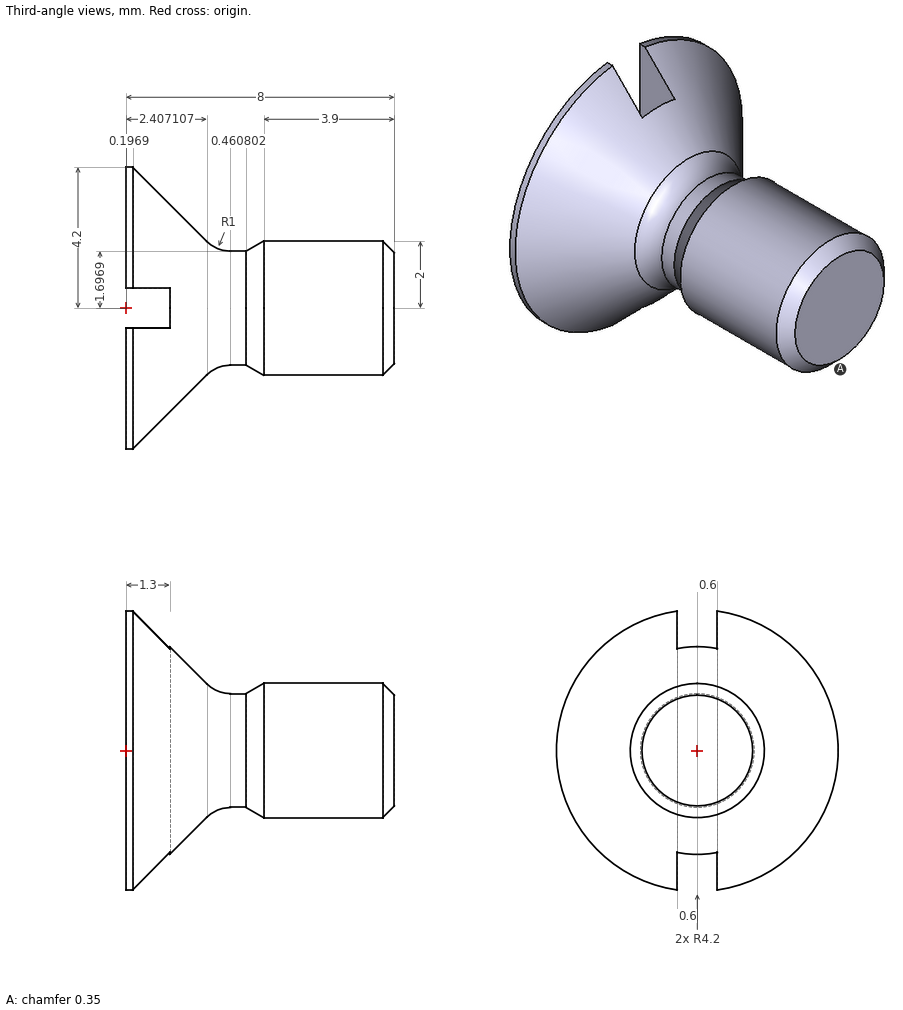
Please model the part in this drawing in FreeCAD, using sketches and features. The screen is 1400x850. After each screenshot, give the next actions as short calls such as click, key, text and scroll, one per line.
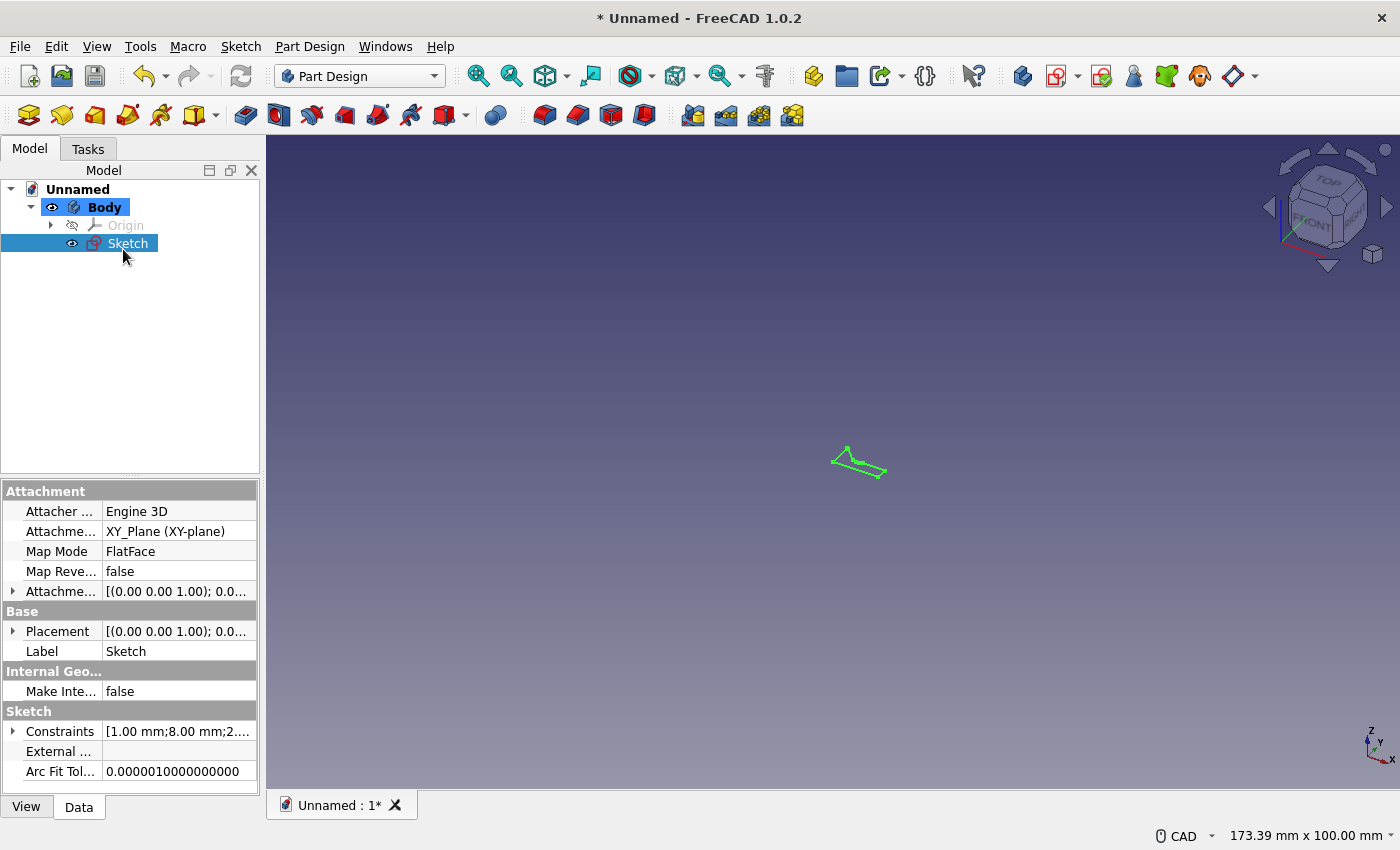
click(62, 116)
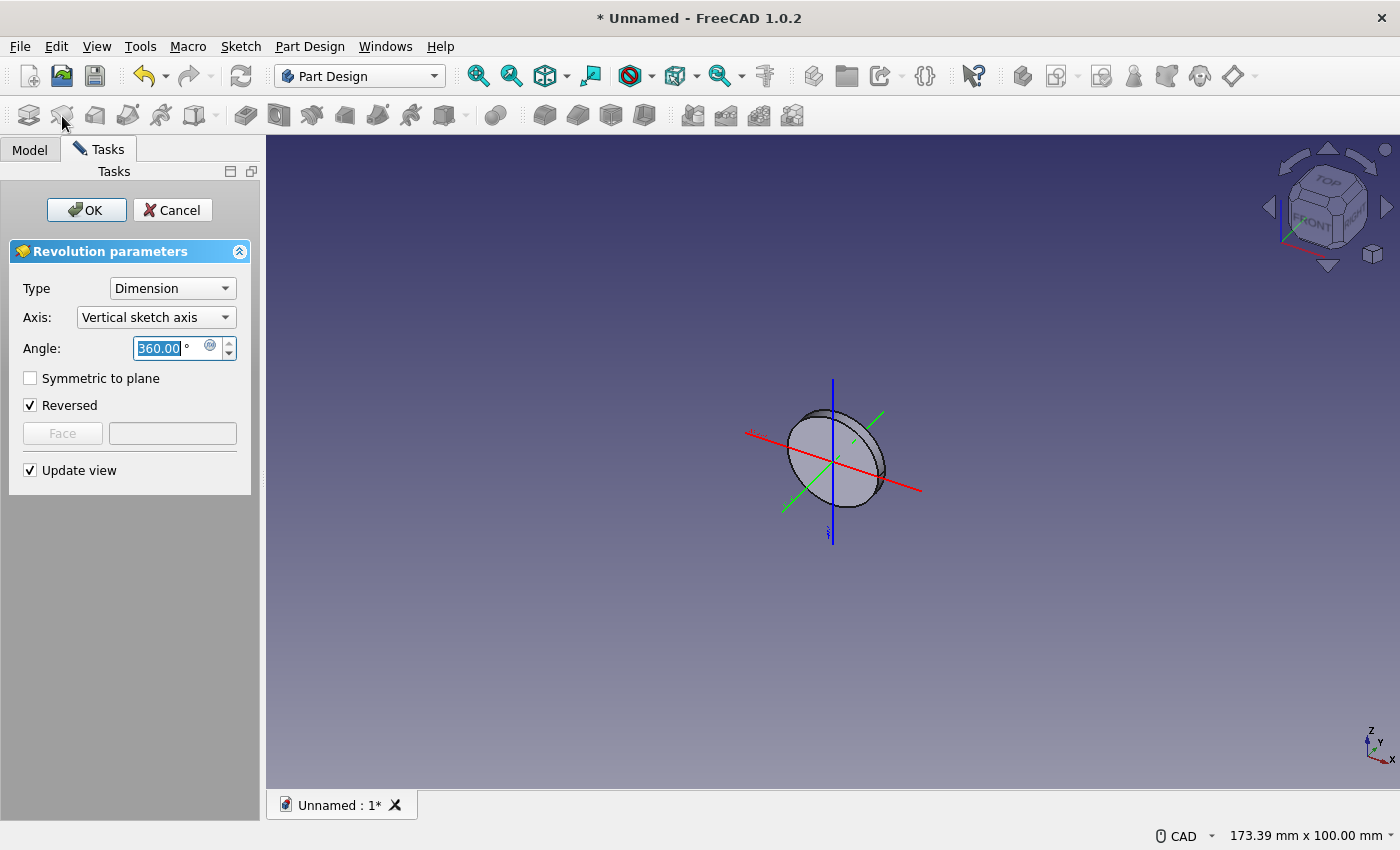
click(157, 318)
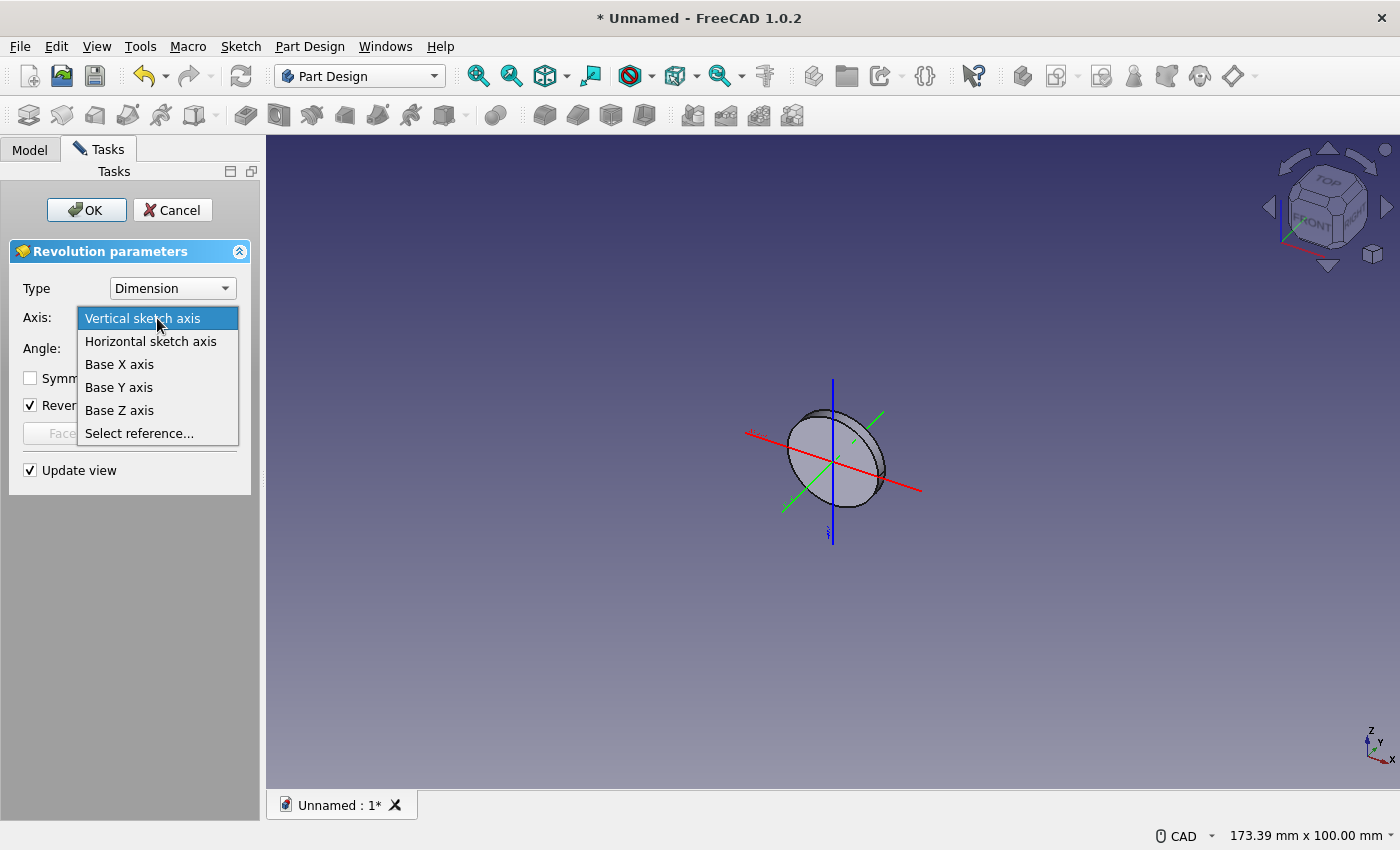
click(156, 342)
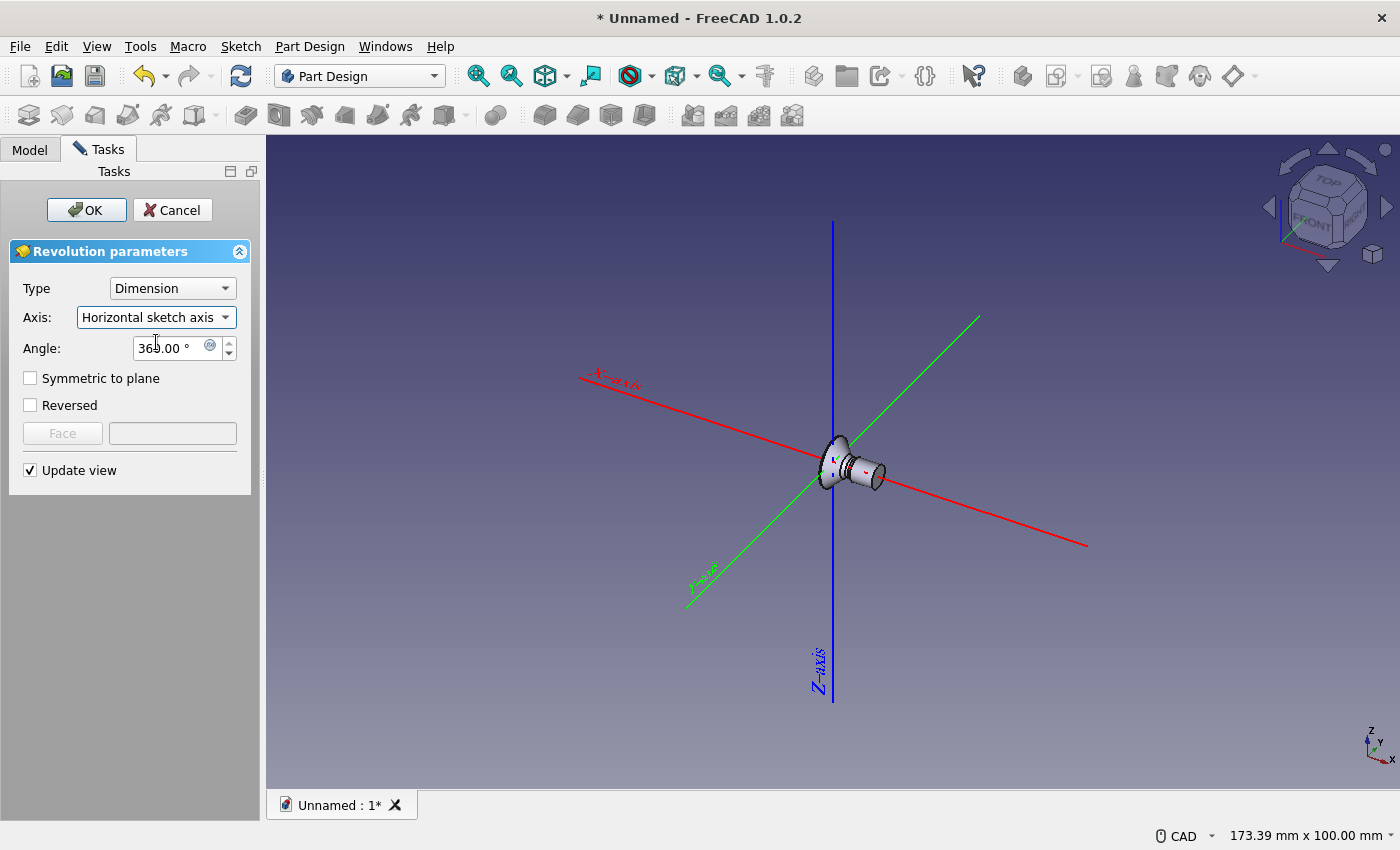
click(87, 210)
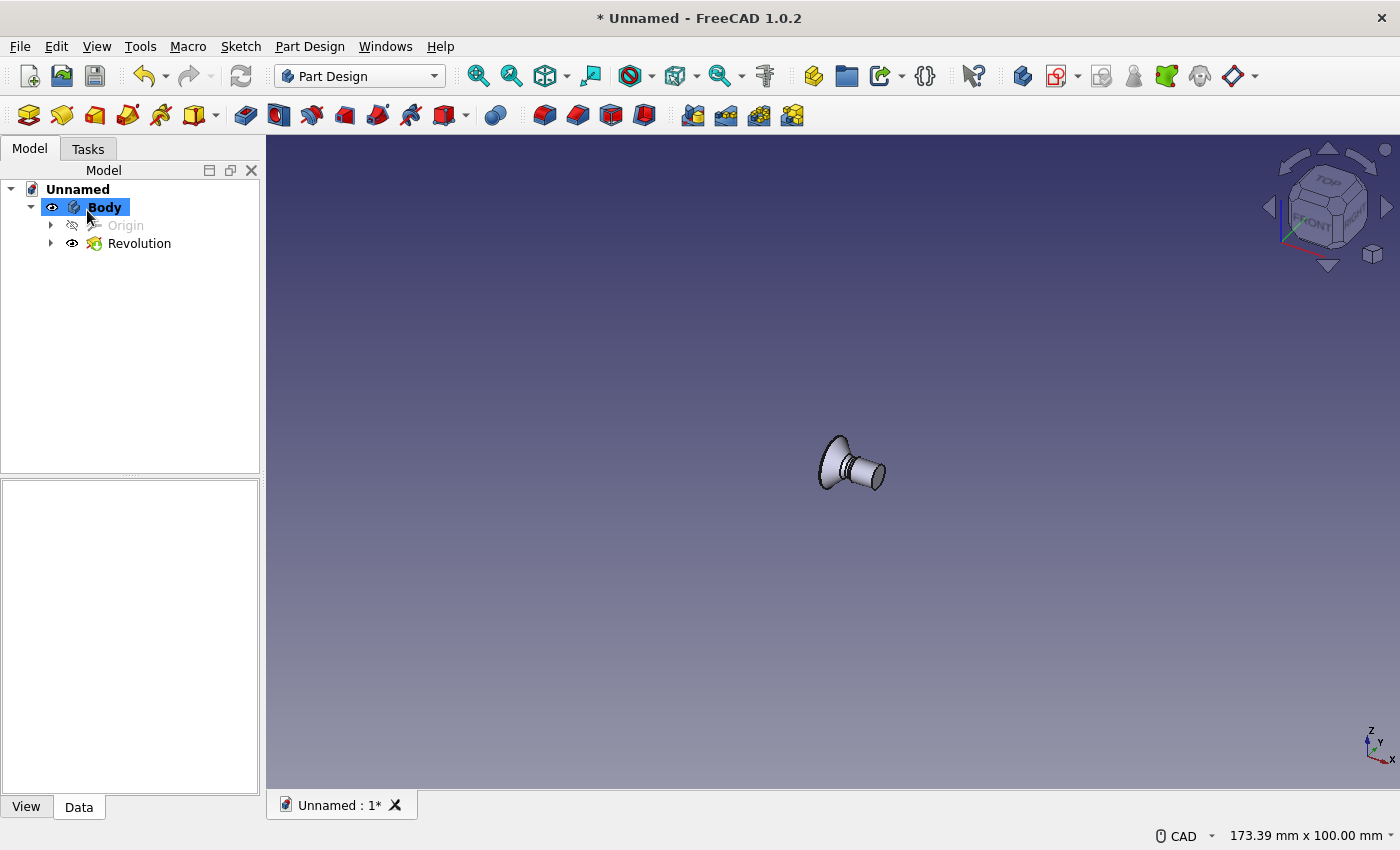
key(v)
key(f)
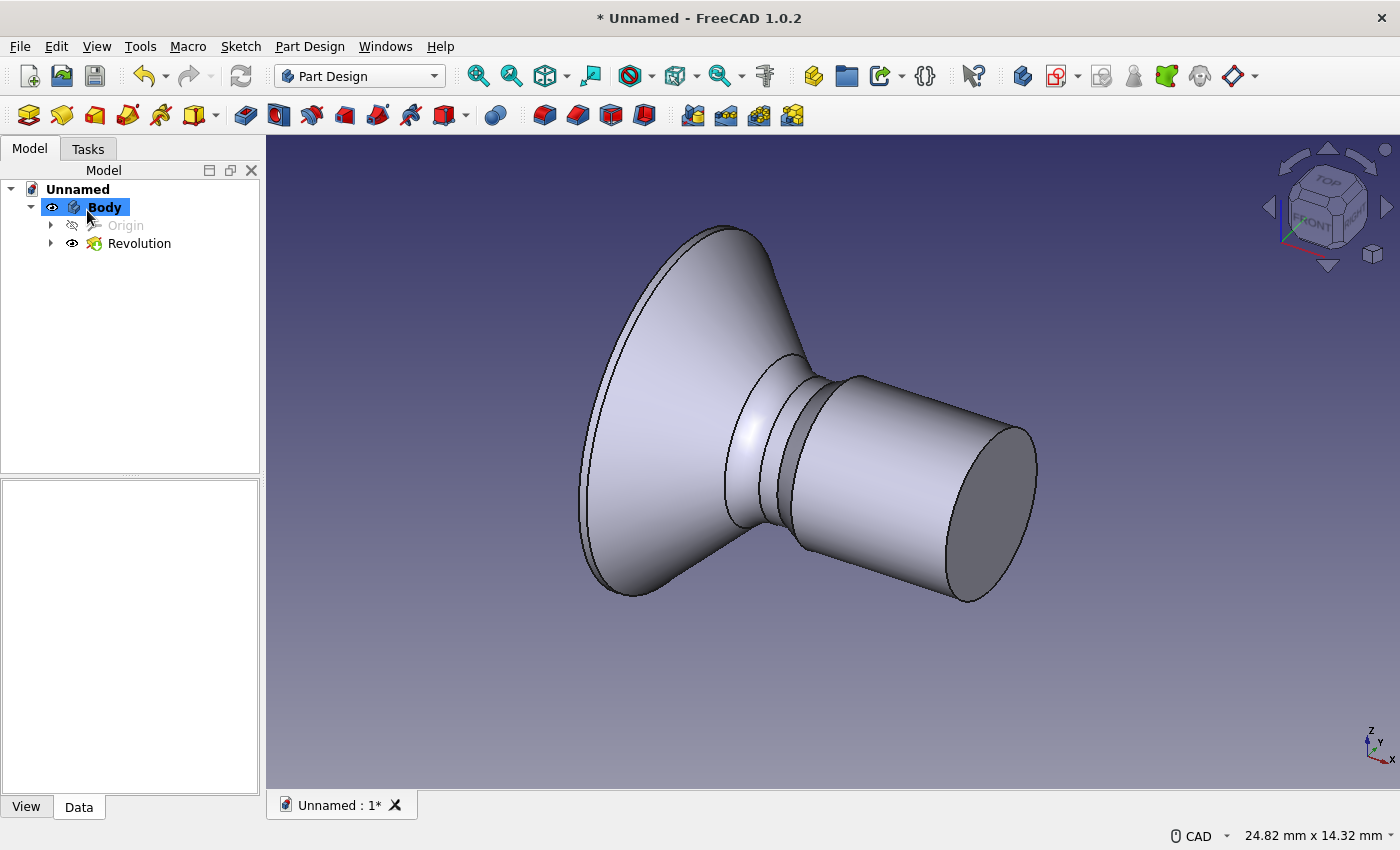
click(945, 559)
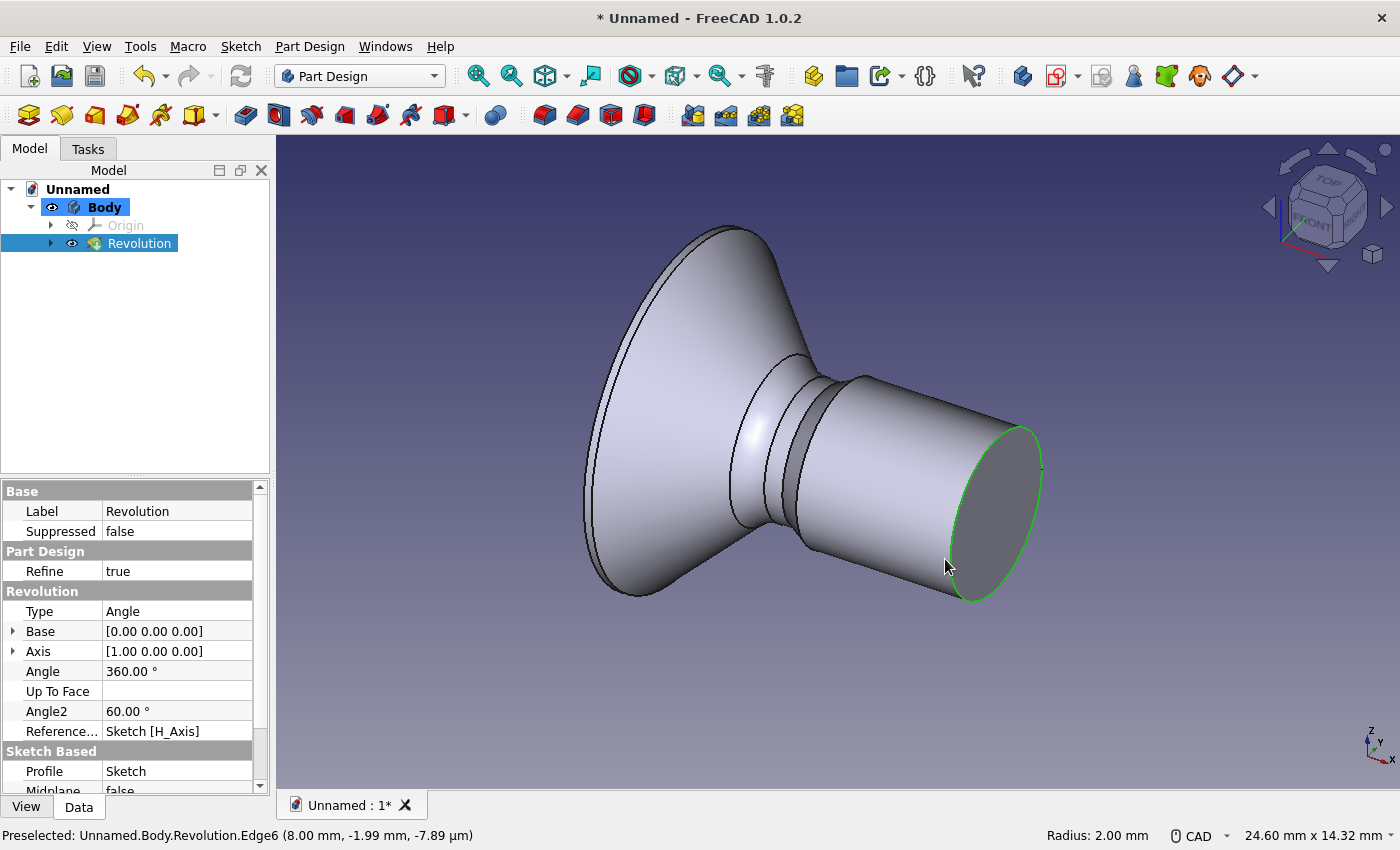
click(578, 116)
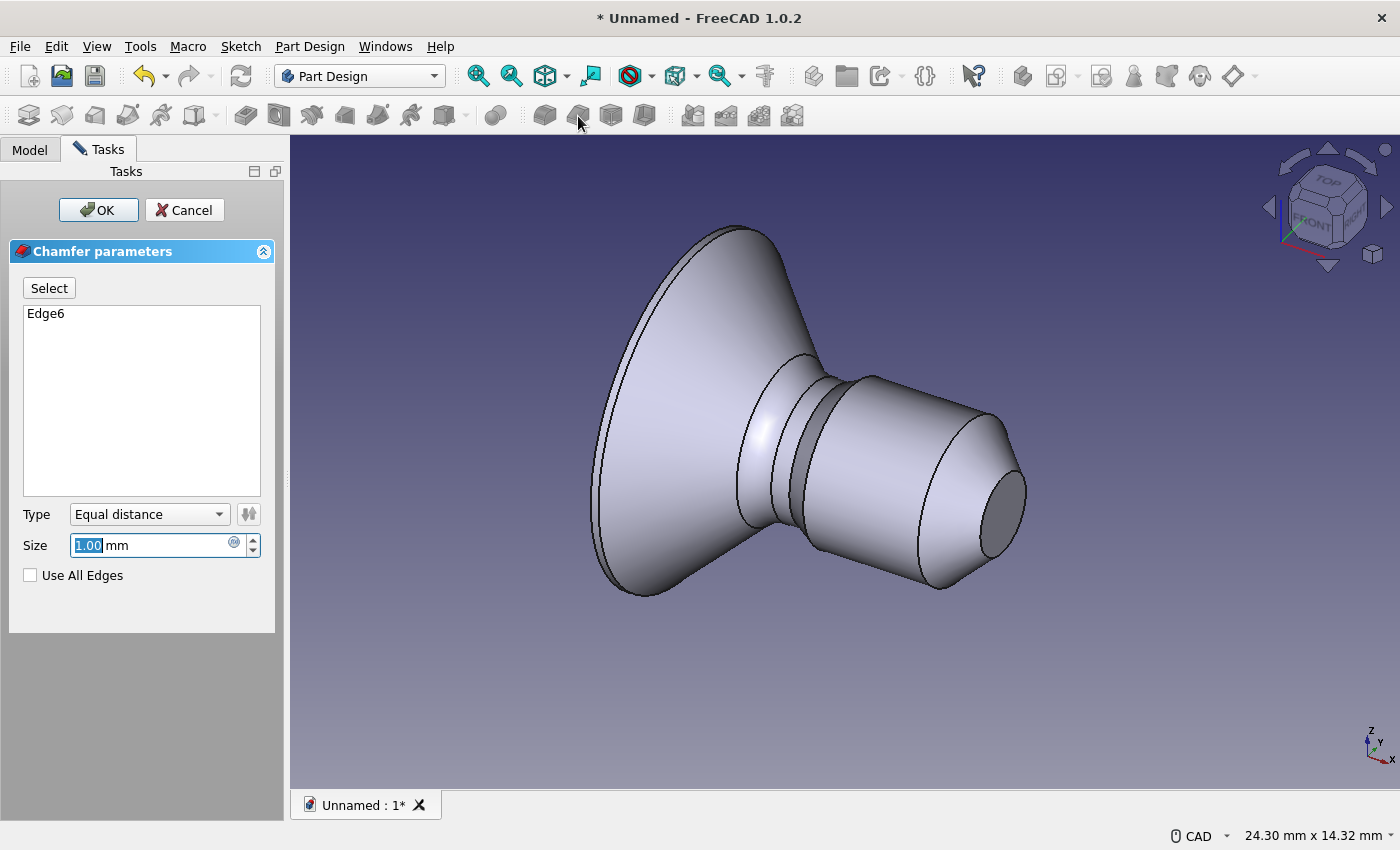
text(0.35)
key(Tab)